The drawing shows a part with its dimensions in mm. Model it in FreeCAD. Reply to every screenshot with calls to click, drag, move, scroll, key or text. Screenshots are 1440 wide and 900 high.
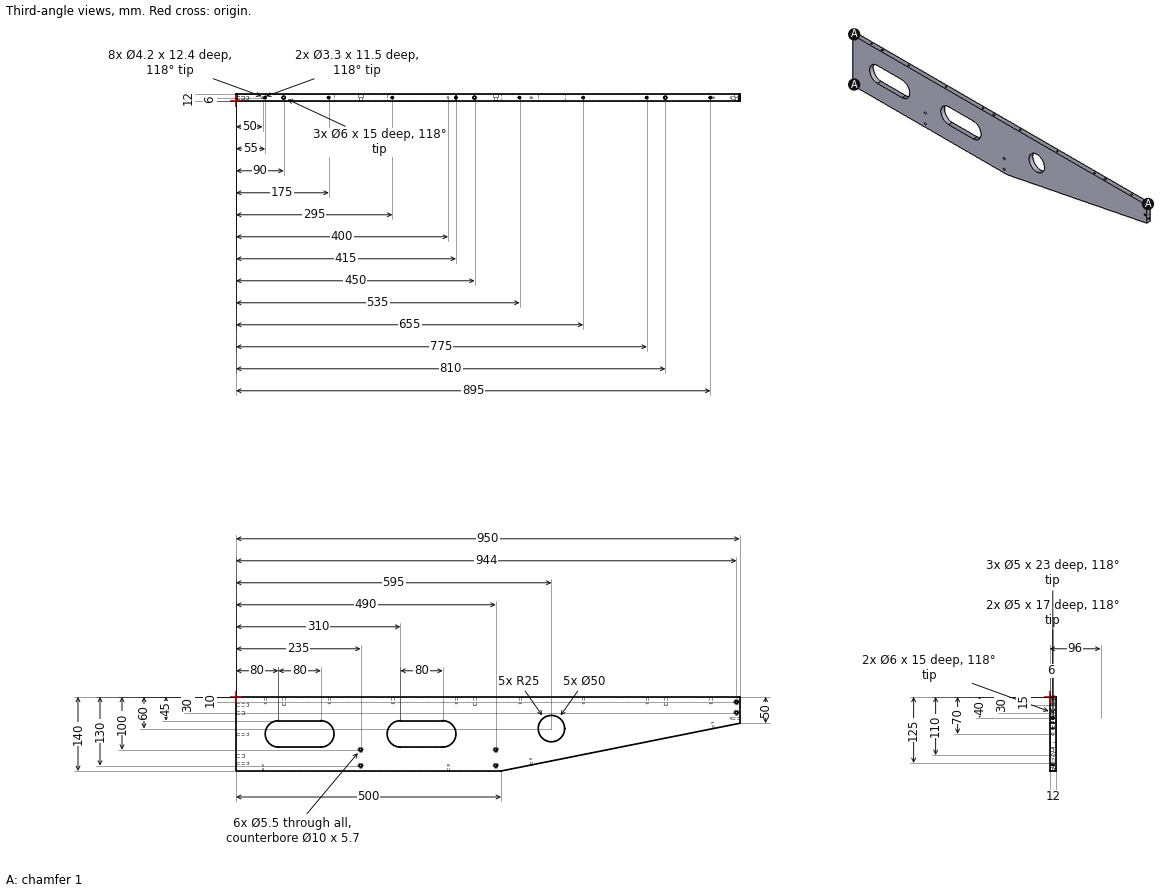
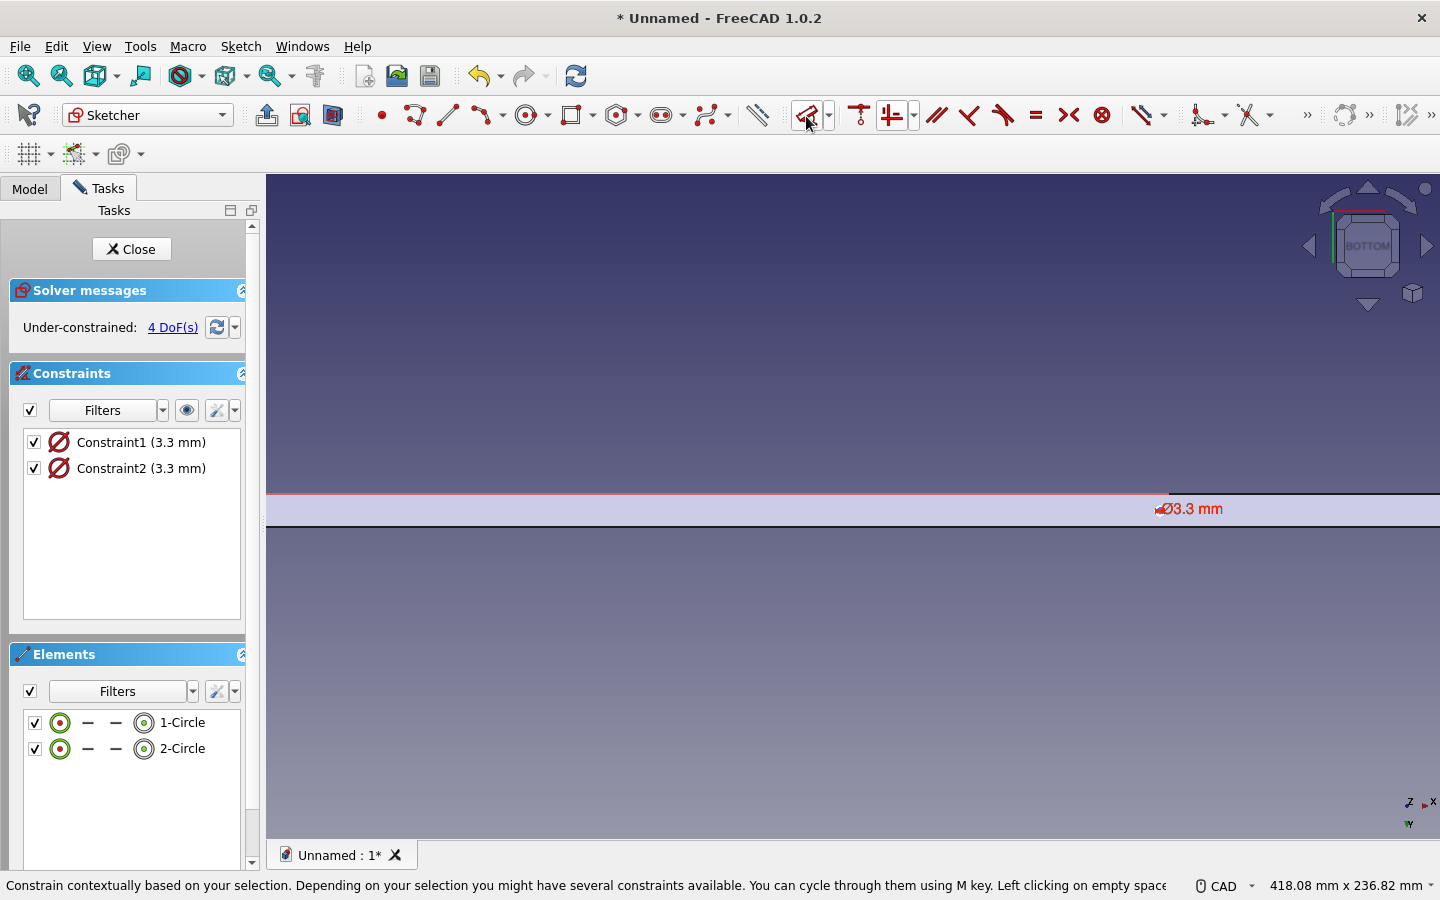
scroll(1158, 511, down, 2)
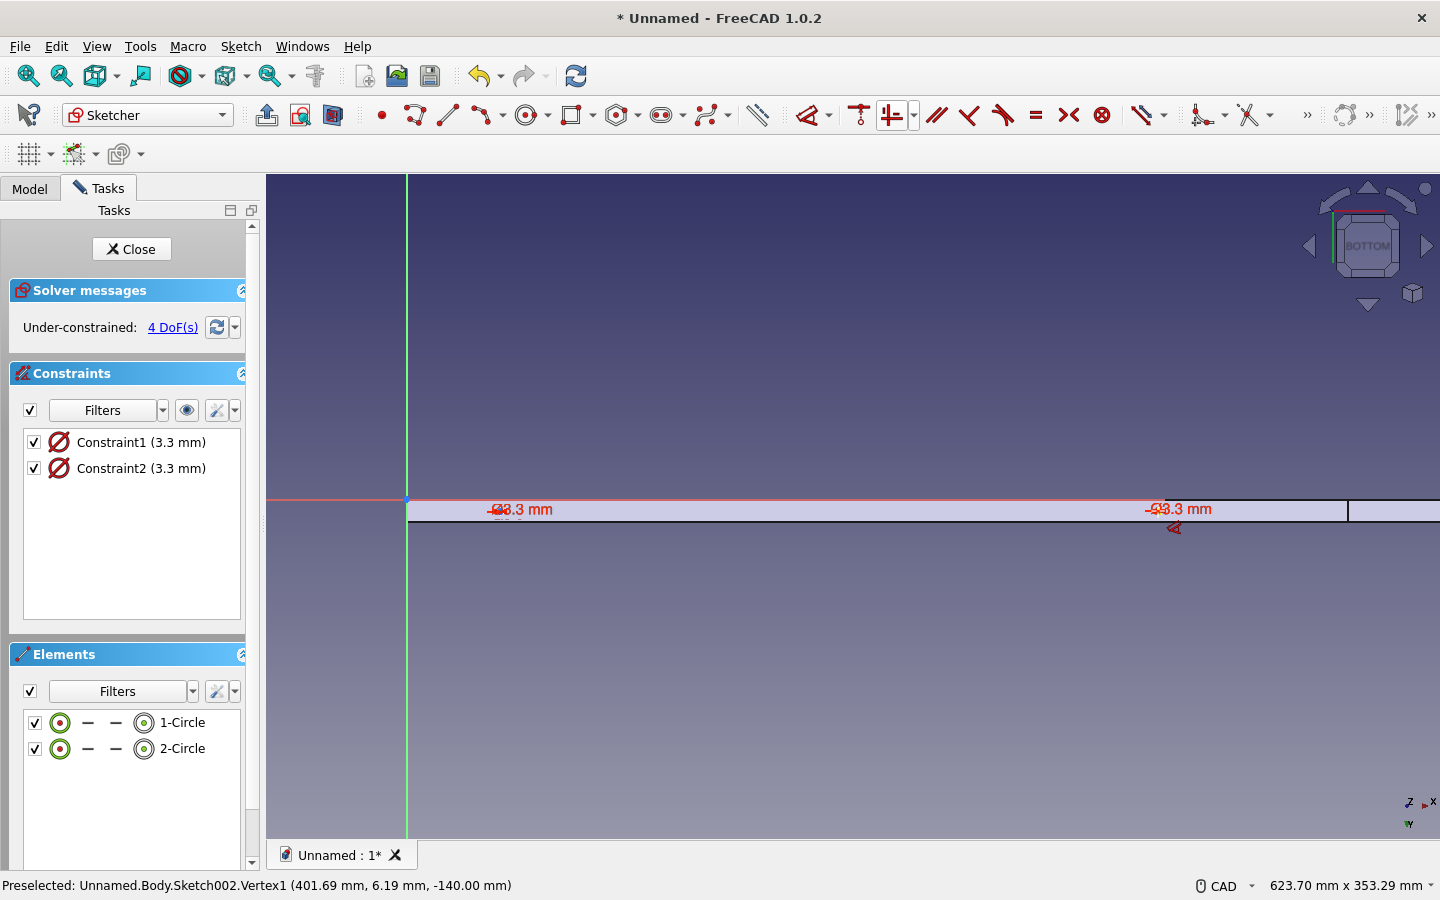
scroll(501, 512, up, 7)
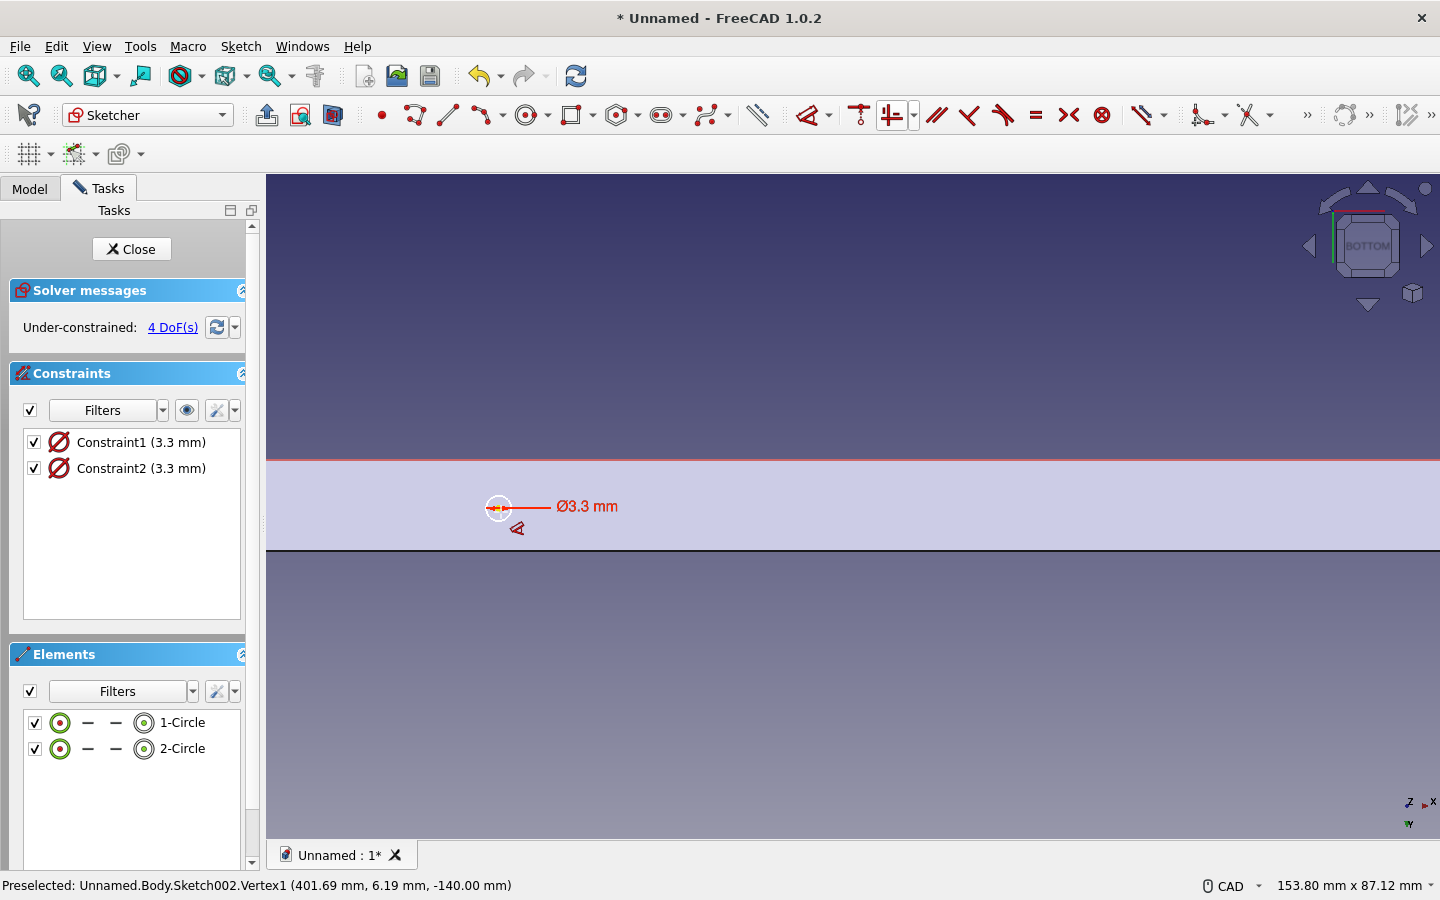
click(499, 508)
click(533, 484)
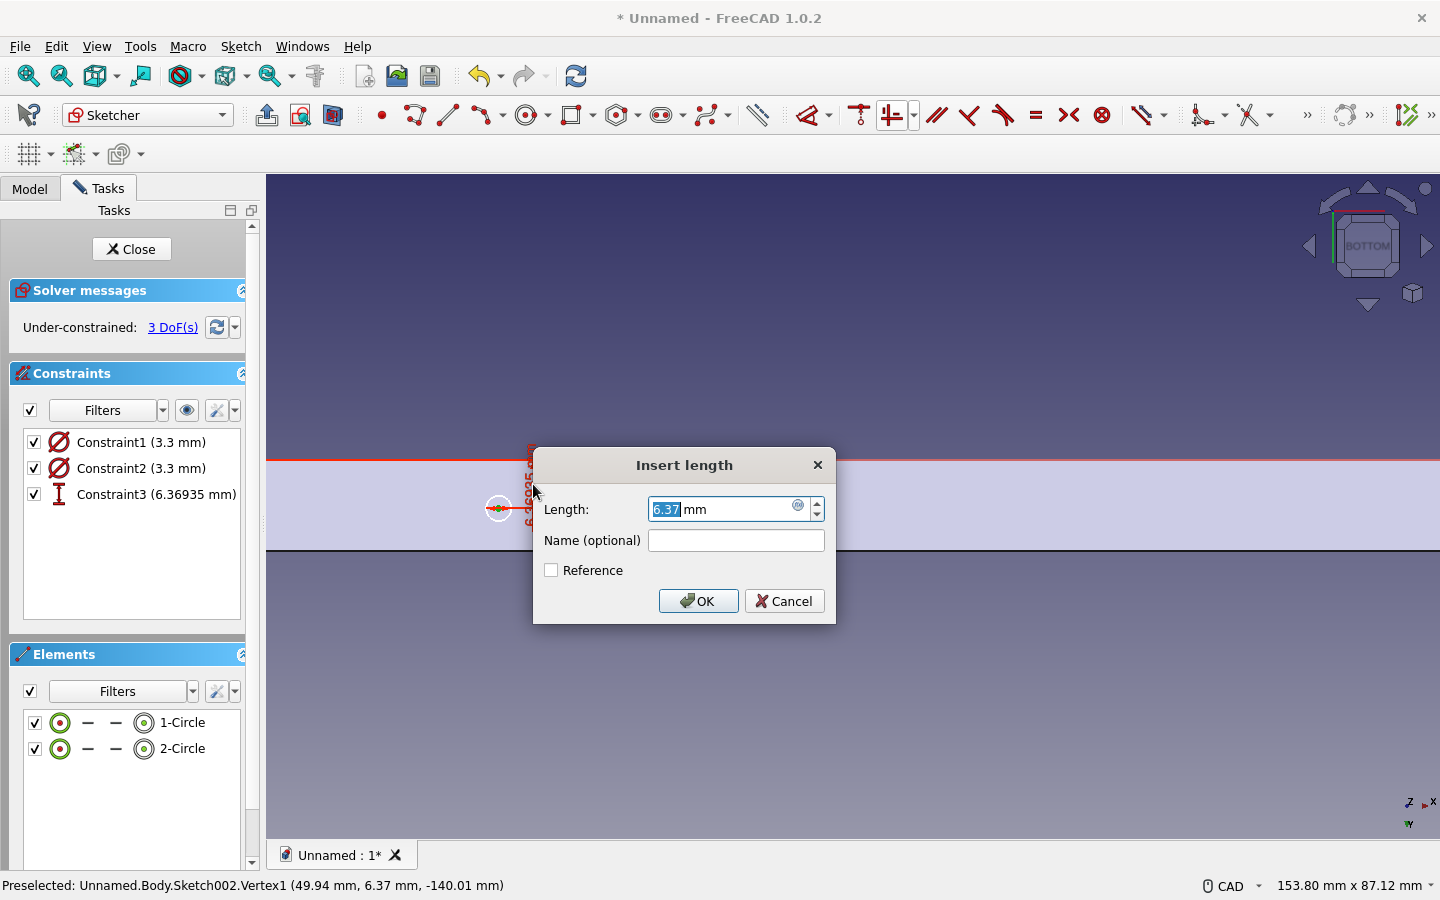
text(6)
key(Return)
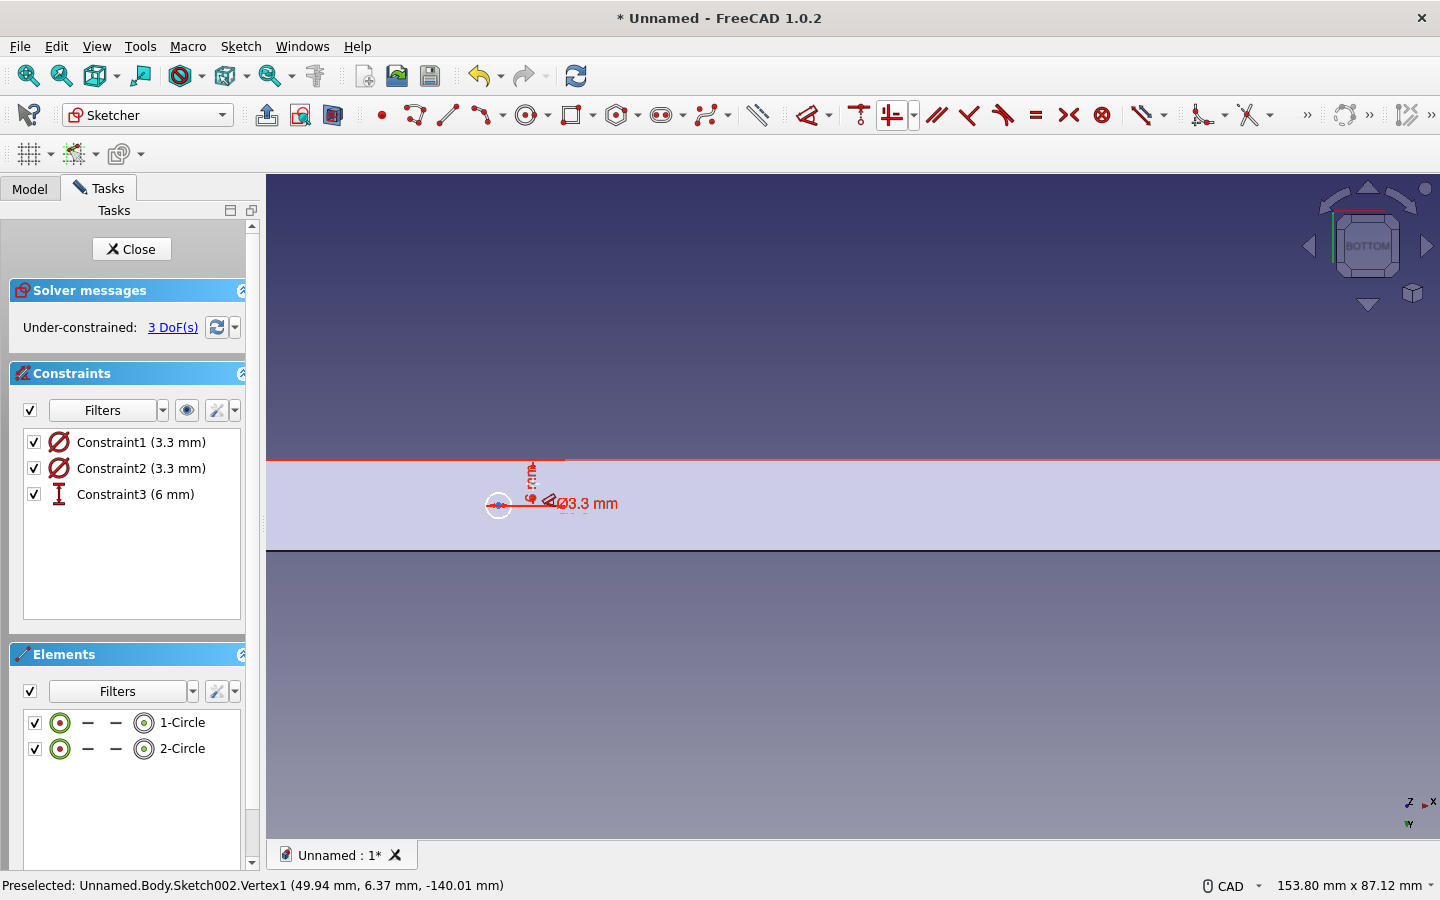
scroll(501, 512, down, 7)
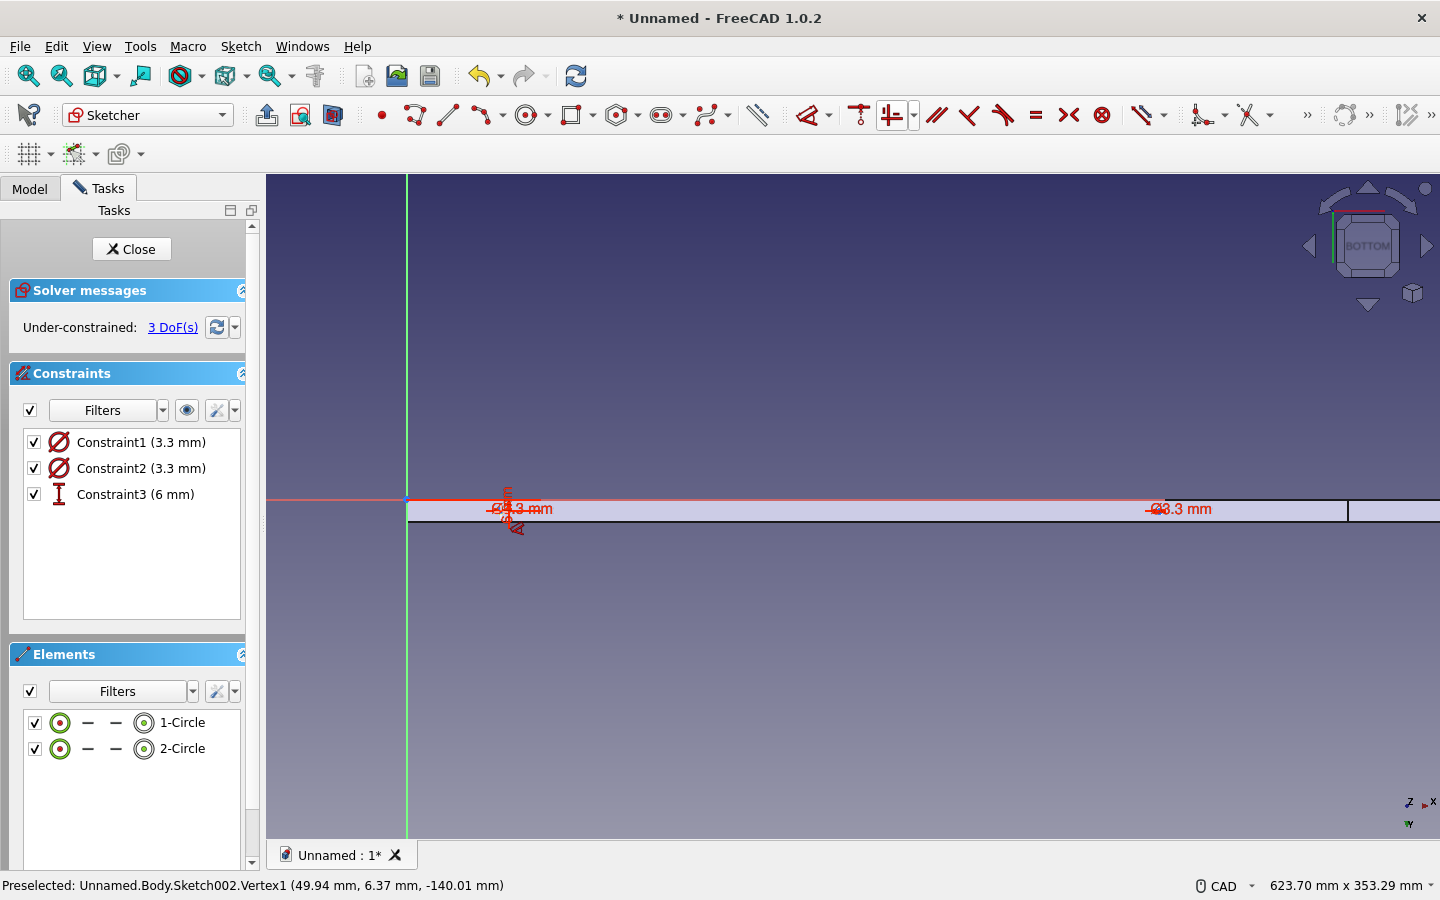
scroll(1160, 511, up, 7)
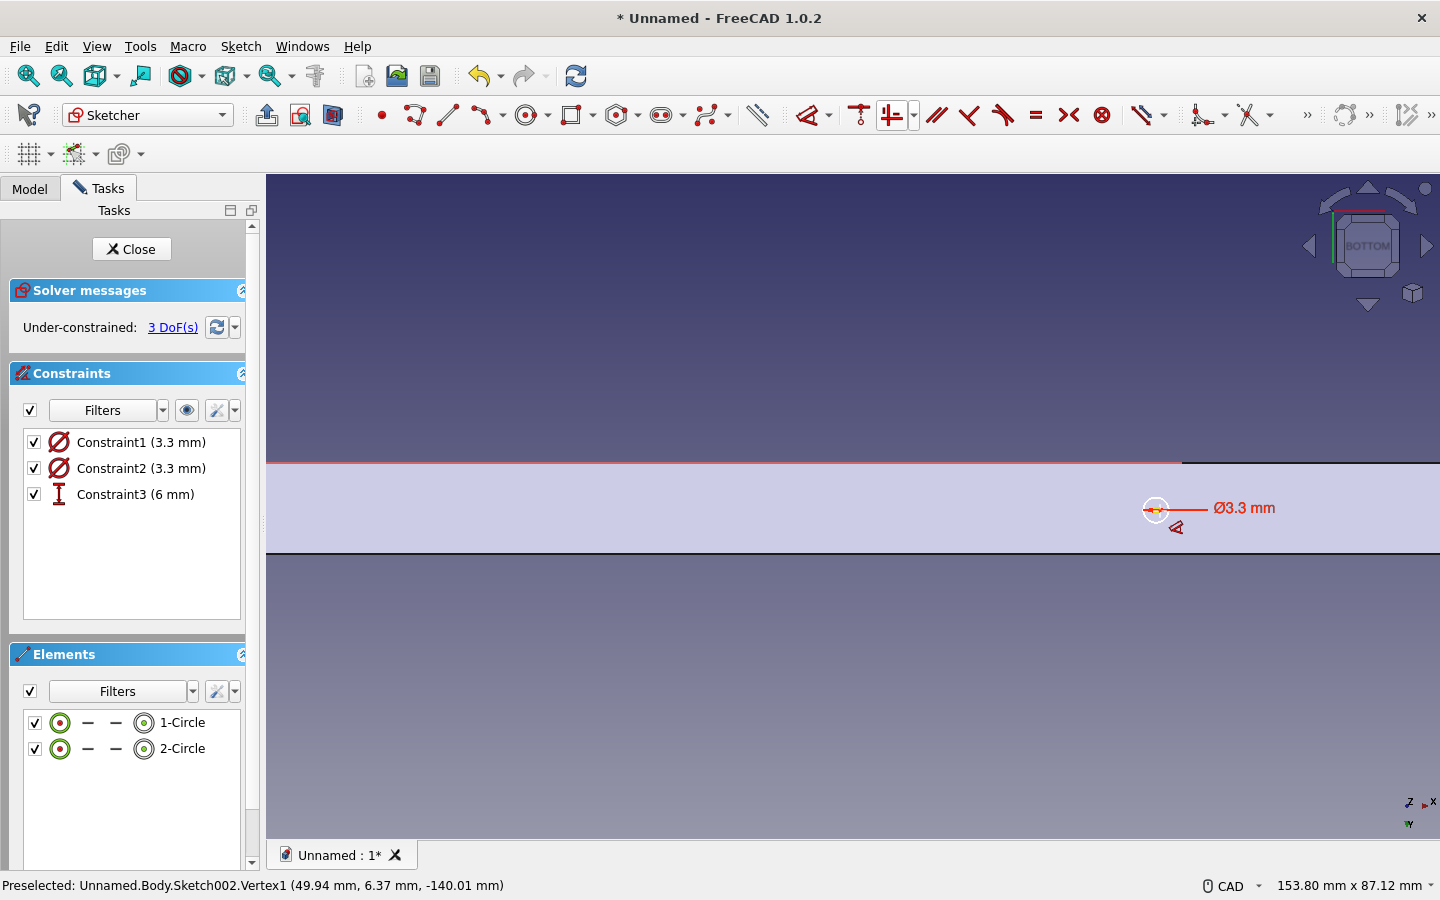
click(1156, 510)
click(1190, 487)